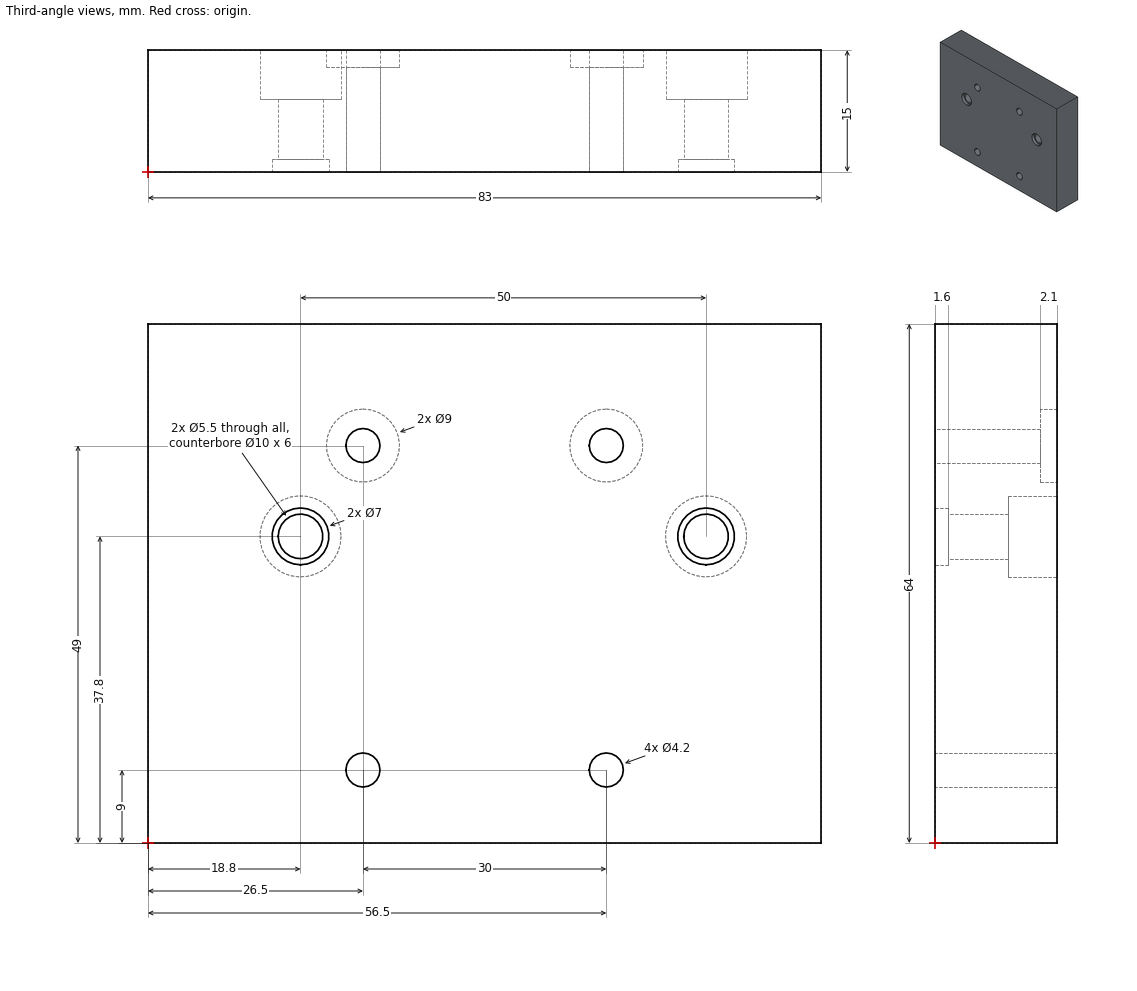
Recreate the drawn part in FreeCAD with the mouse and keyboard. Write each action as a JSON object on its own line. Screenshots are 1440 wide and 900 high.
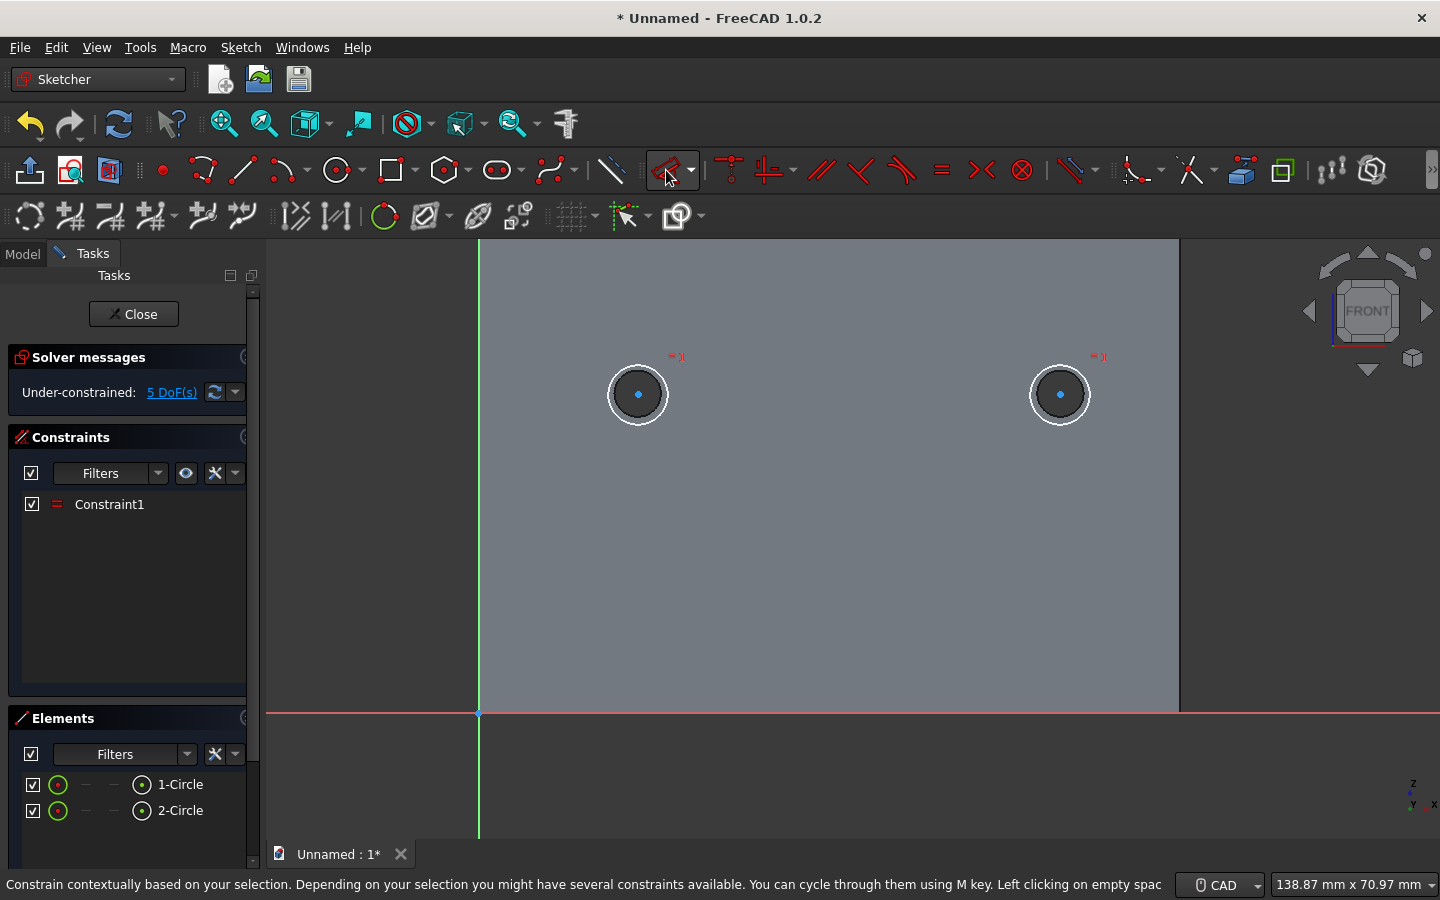
{"action": "left_click", "coordinate": [659, 374]}
{"action": "left_click", "coordinate": [682, 351]}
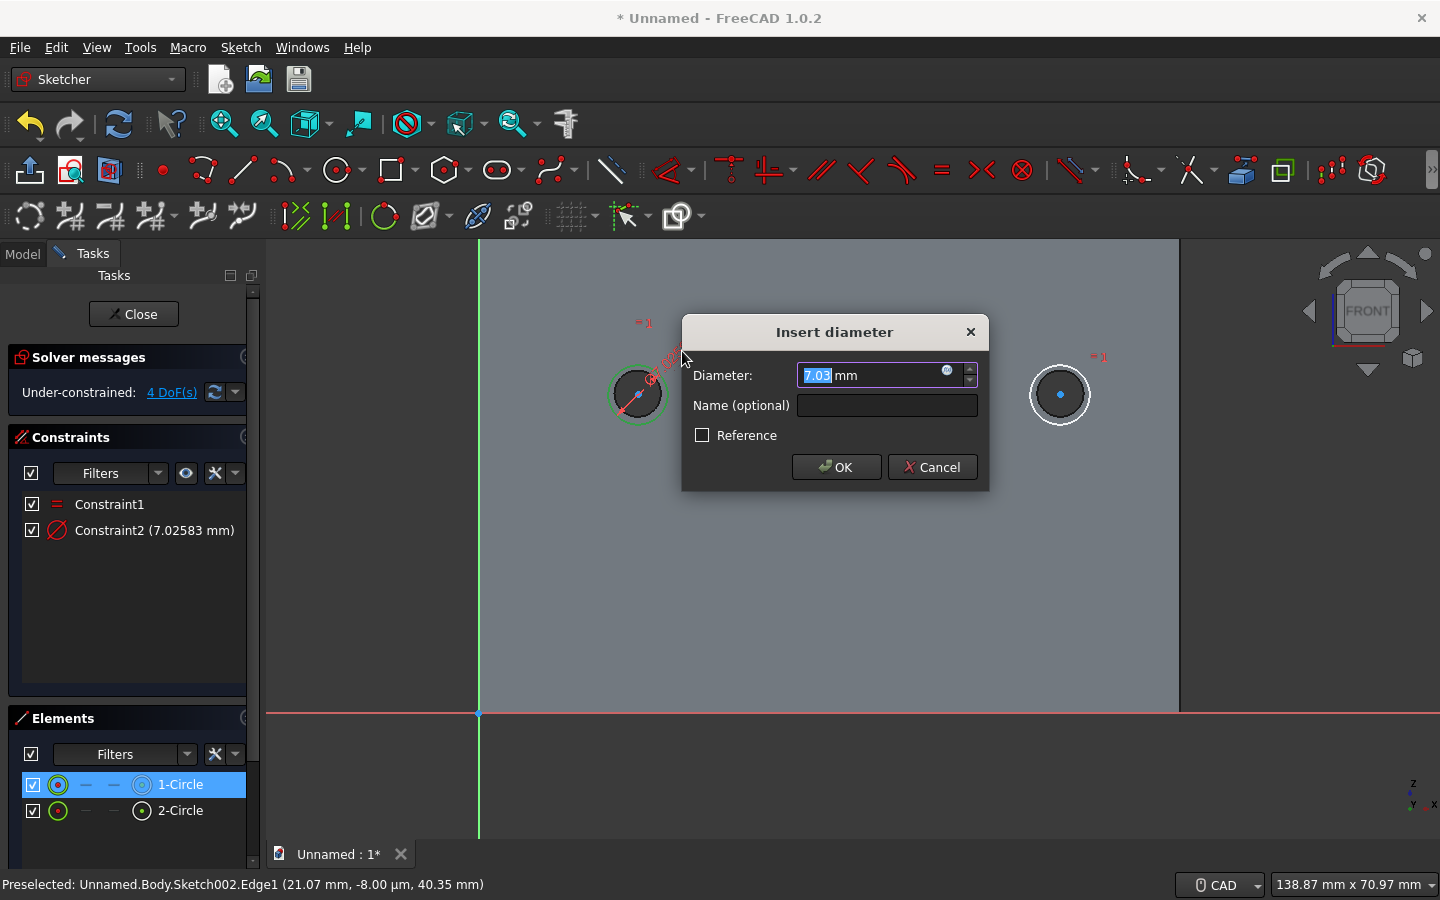
{"action": "type", "text": "7"}
{"action": "key", "text": "Return"}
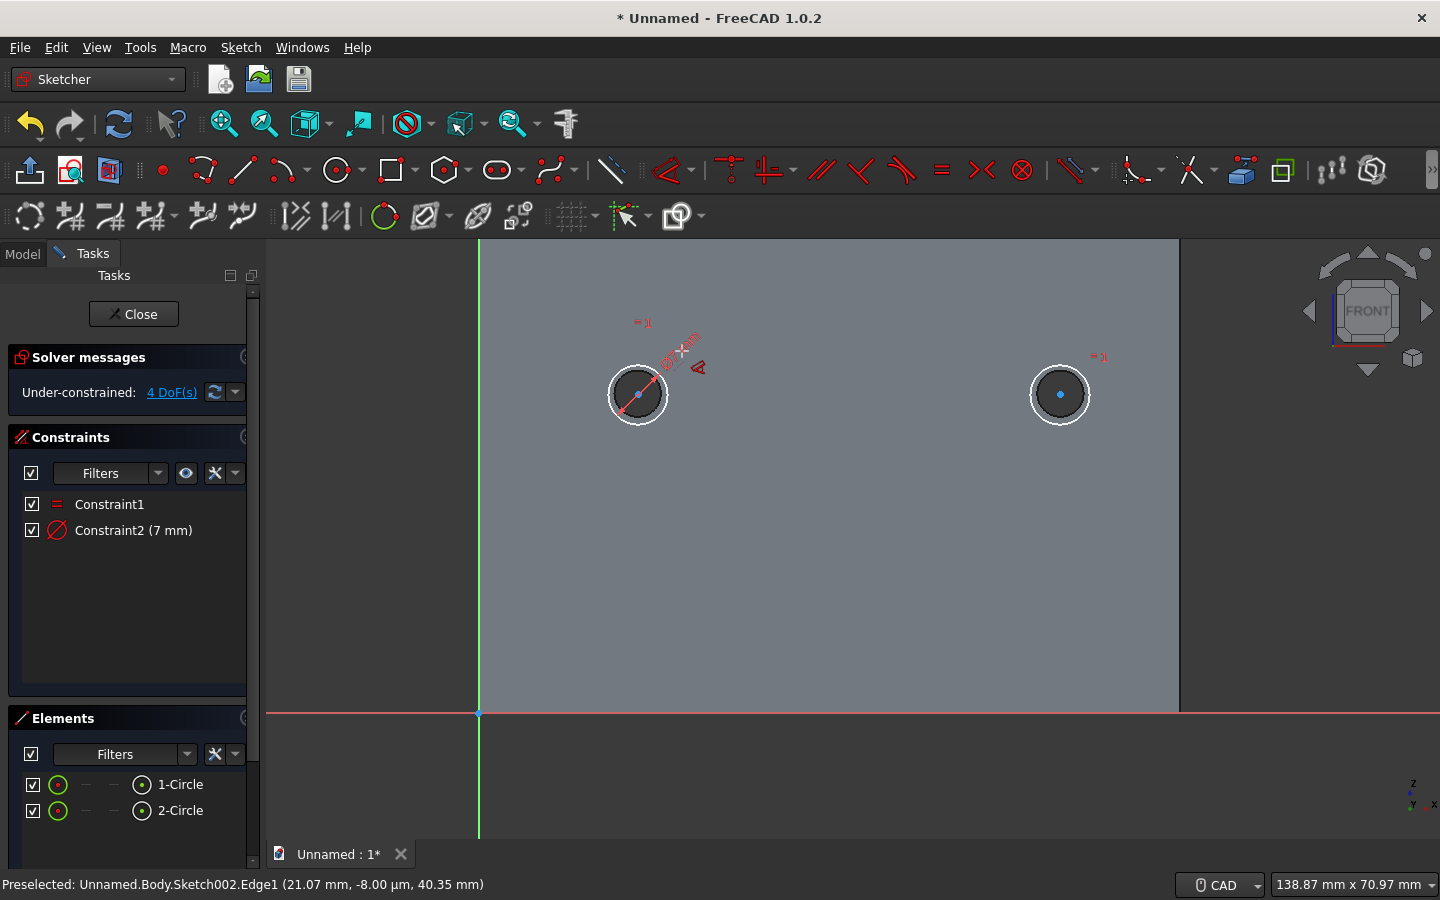
{"action": "left_click", "coordinate": [638, 395]}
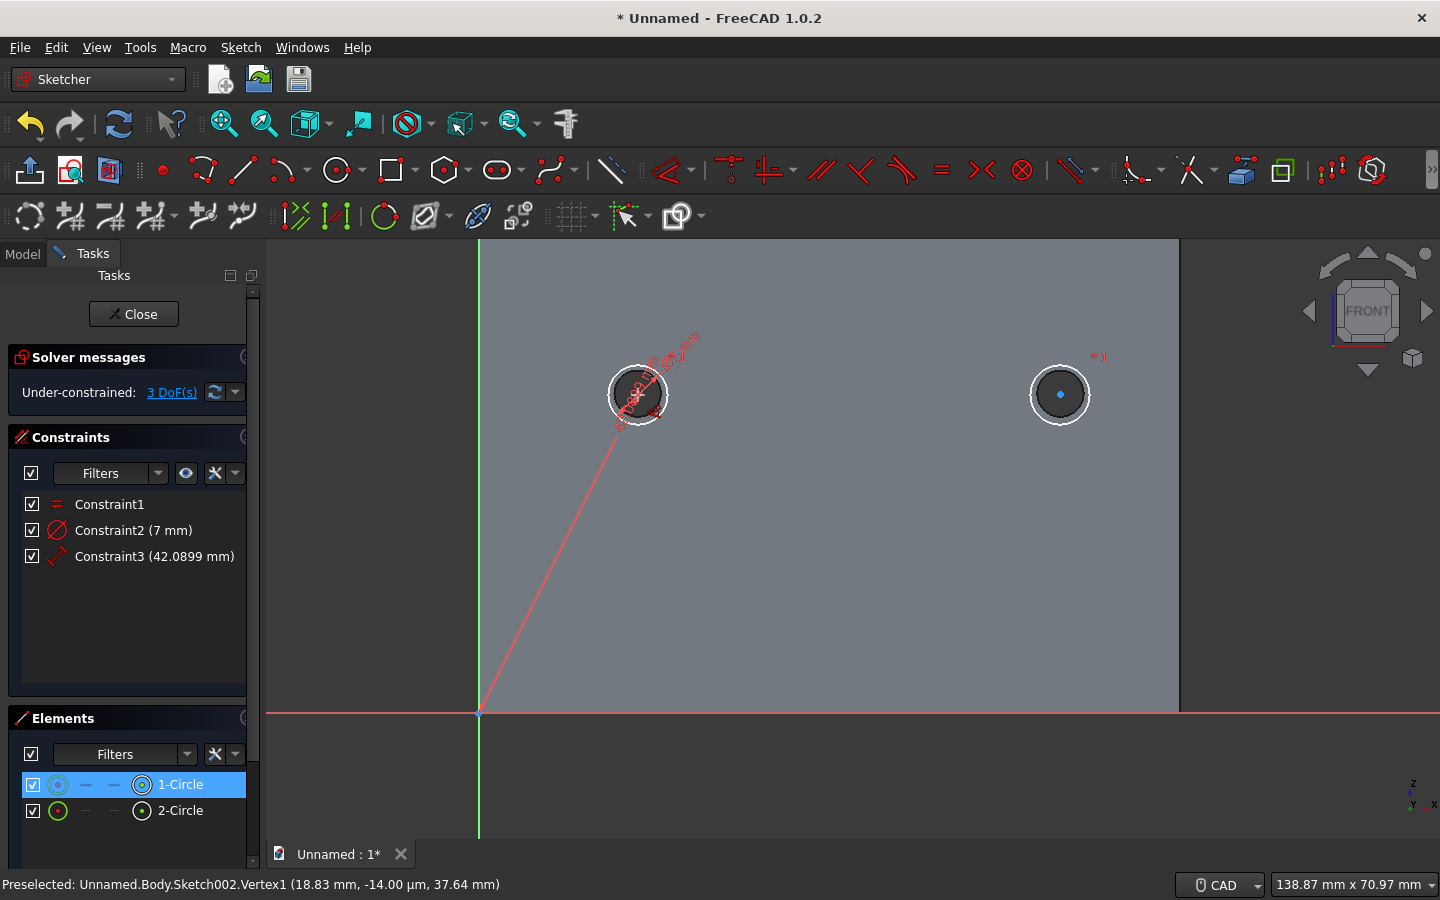
{"action": "left_click", "coordinate": [1060, 395]}
{"action": "left_click", "coordinate": [849, 361]}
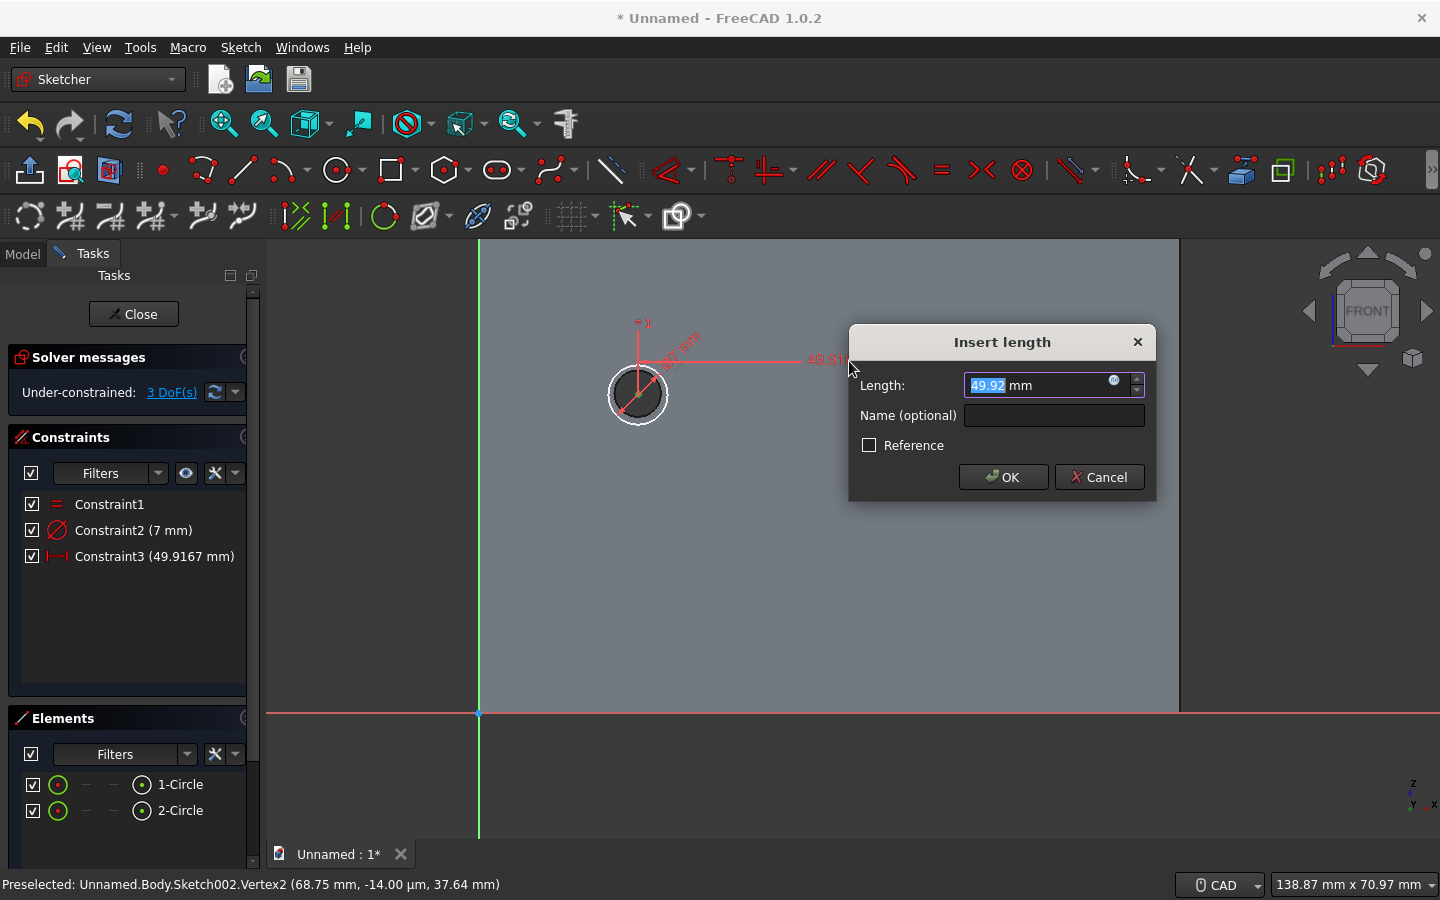
{"action": "type", "text": "50"}
{"action": "key", "text": "Return"}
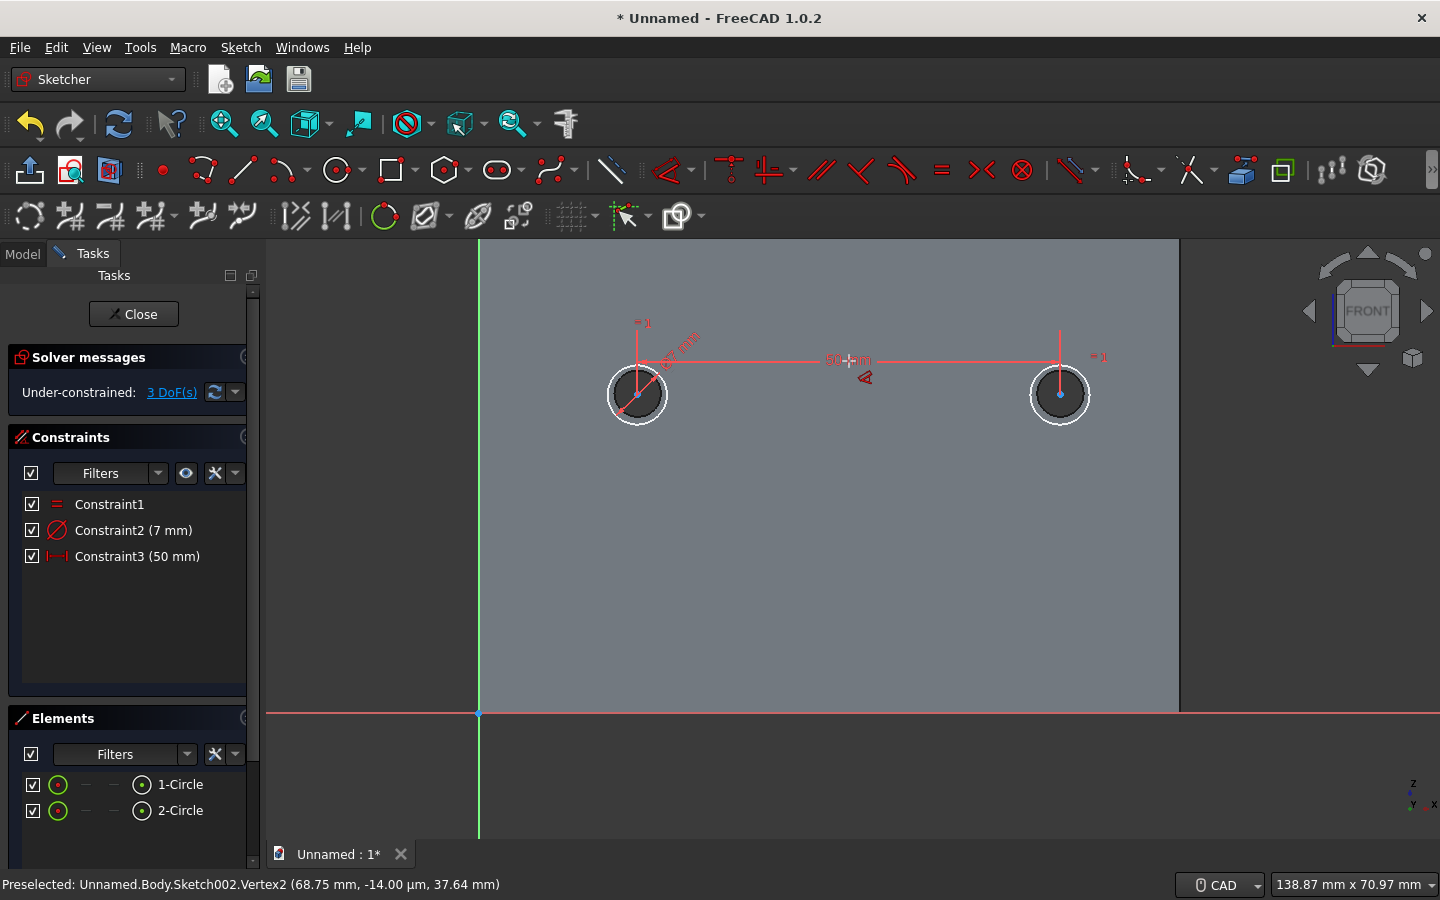
{"action": "left_click", "coordinate": [637, 395]}
{"action": "left_click", "coordinate": [558, 747]}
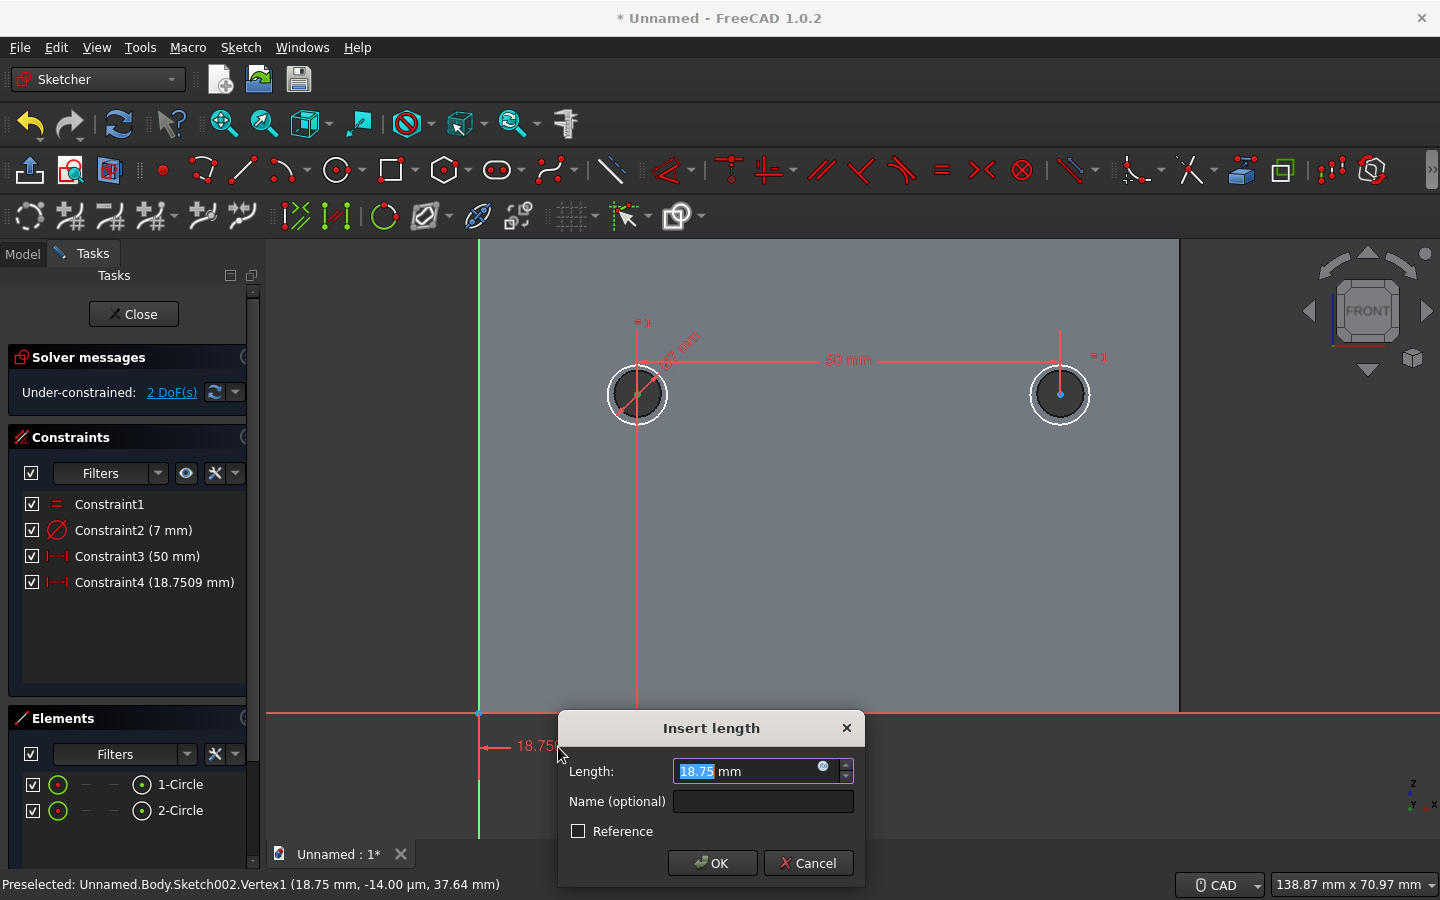
{"action": "type", "text": "18.8"}
{"action": "key", "text": "Return"}